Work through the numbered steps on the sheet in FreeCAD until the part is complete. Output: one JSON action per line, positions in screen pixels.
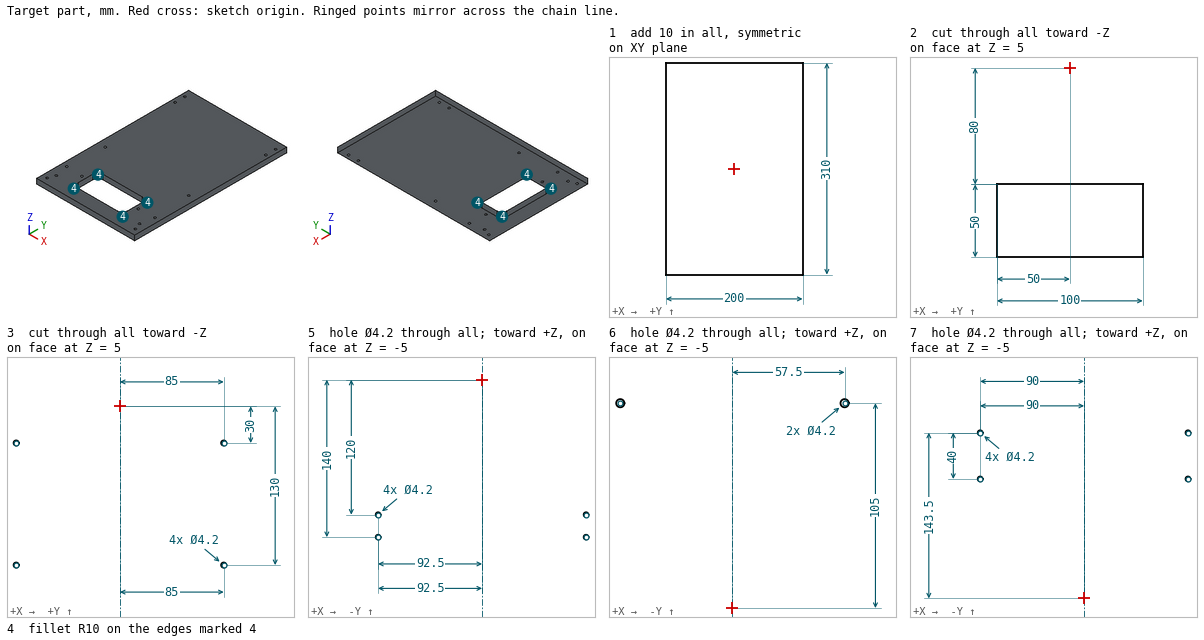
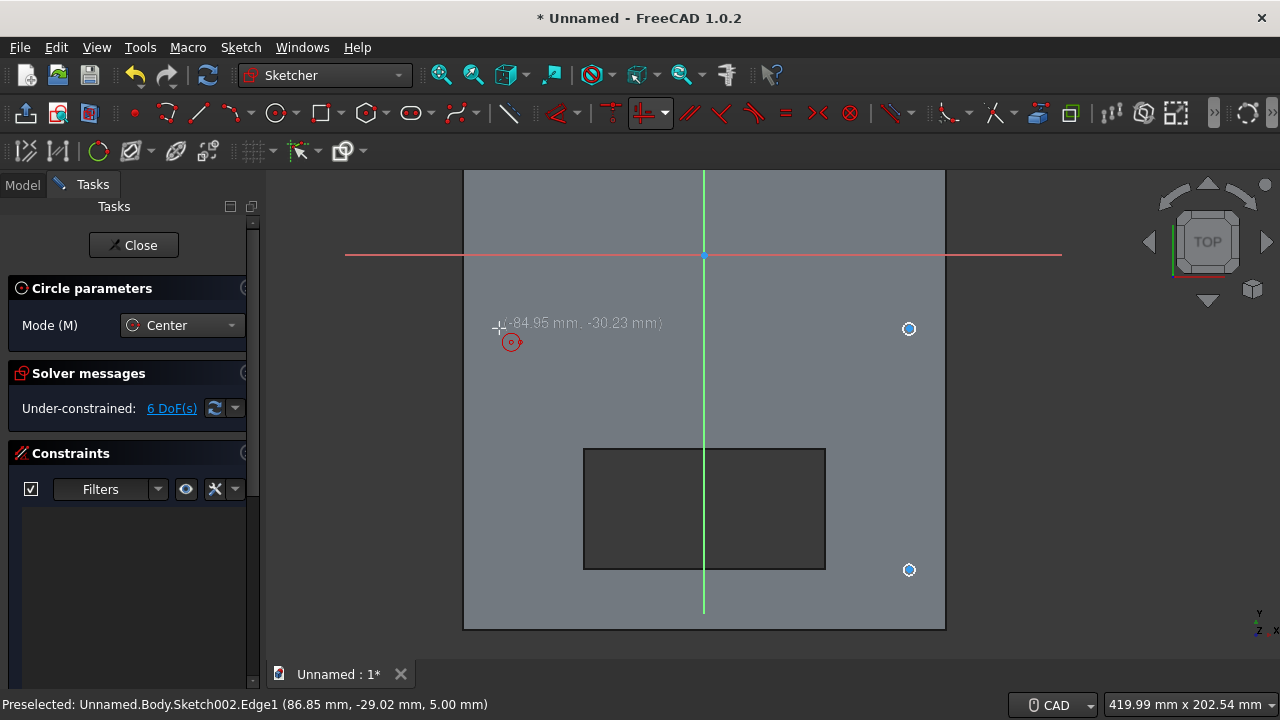
{"action": "left_click", "coordinate": [499, 328]}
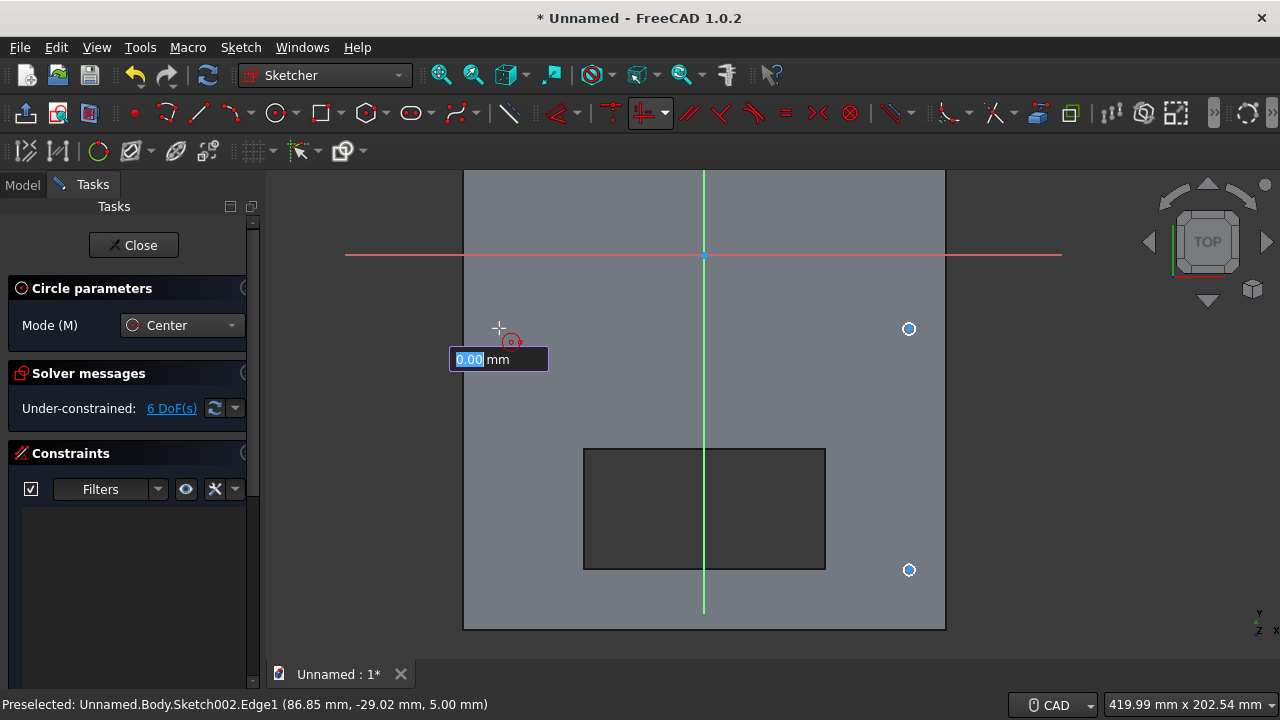
{"action": "scroll", "coordinate": [503, 324], "scroll_direction": "up", "scroll_amount": 6}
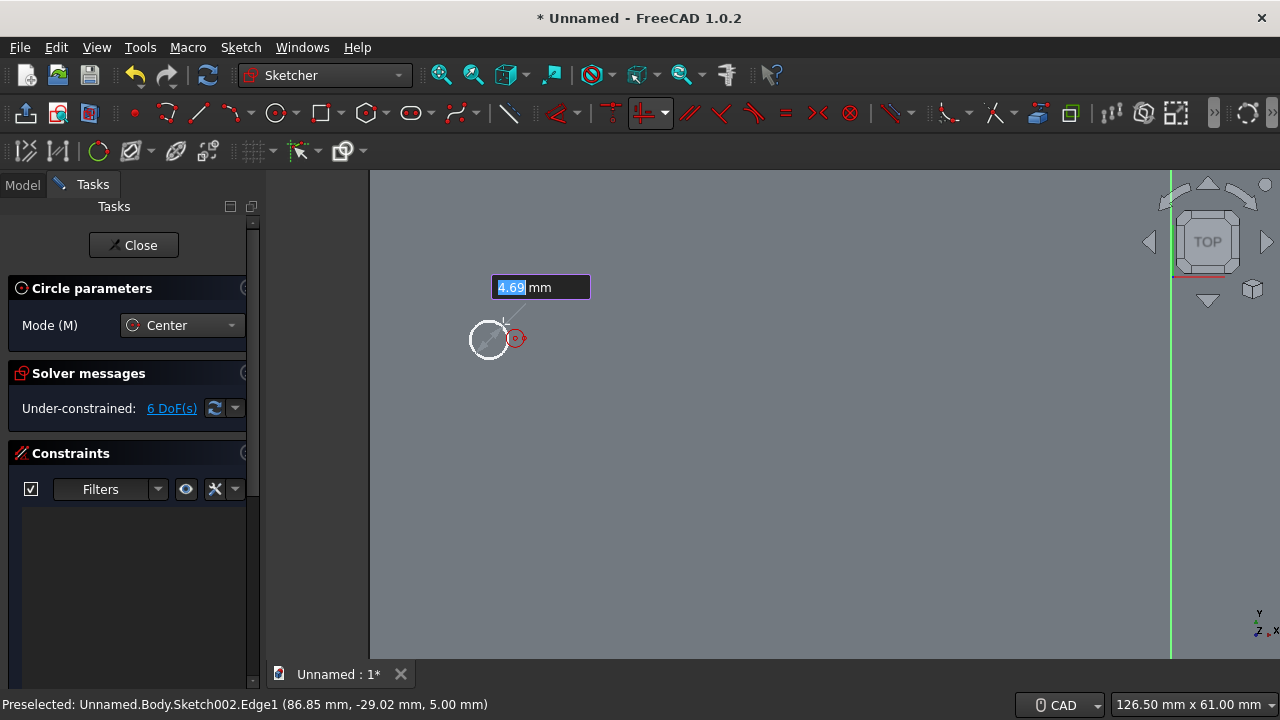
{"action": "left_click", "coordinate": [501, 324]}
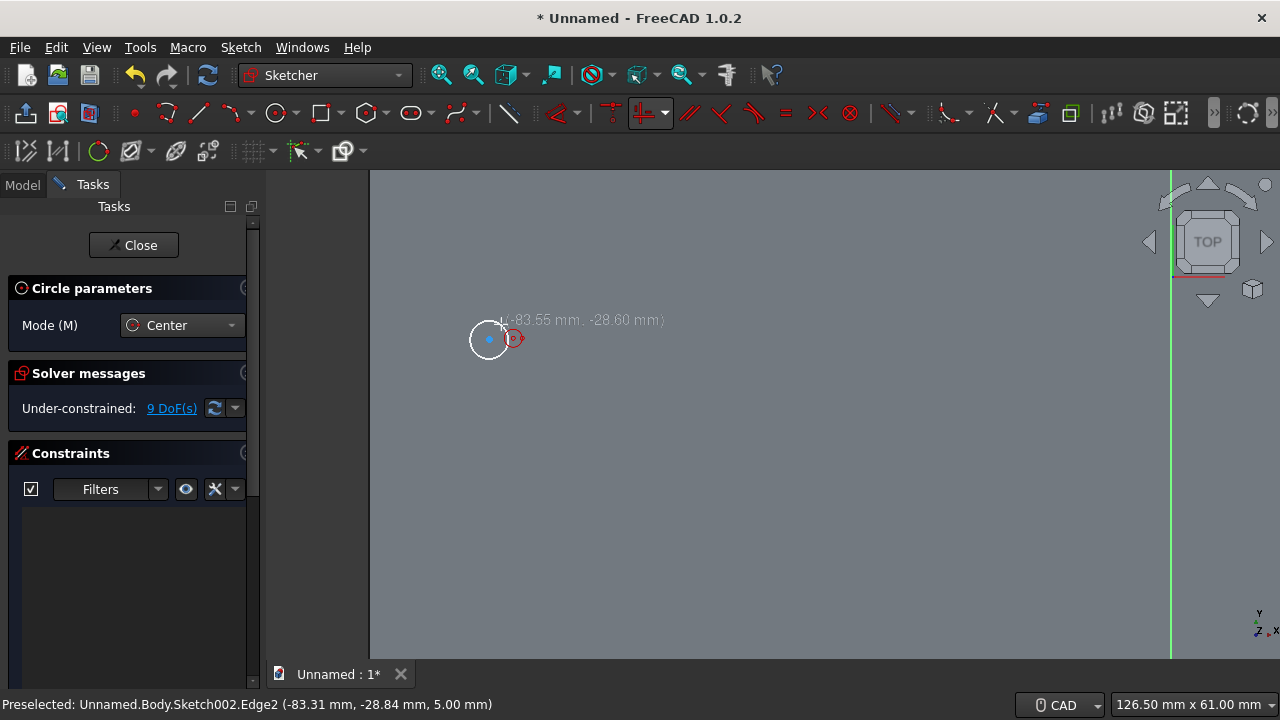
{"action": "scroll", "coordinate": [504, 324], "scroll_direction": "down", "scroll_amount": 6}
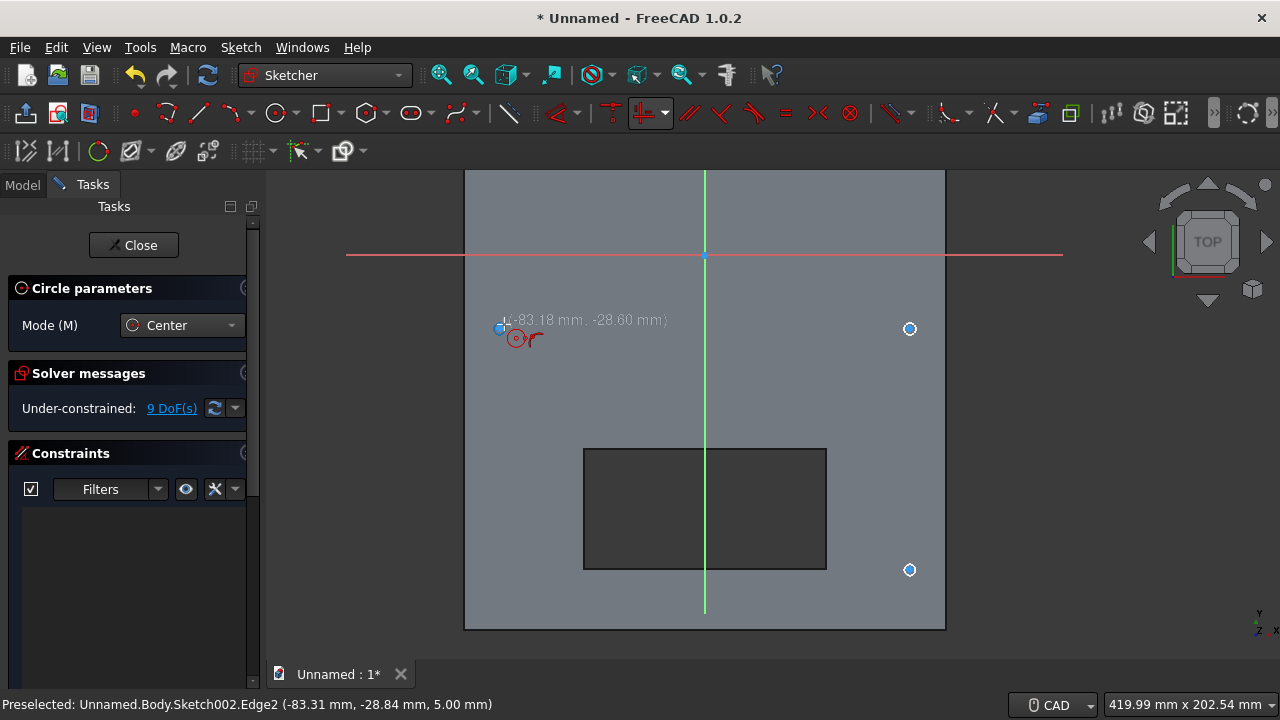
{"action": "scroll", "coordinate": [500, 569], "scroll_direction": "up", "scroll_amount": 8}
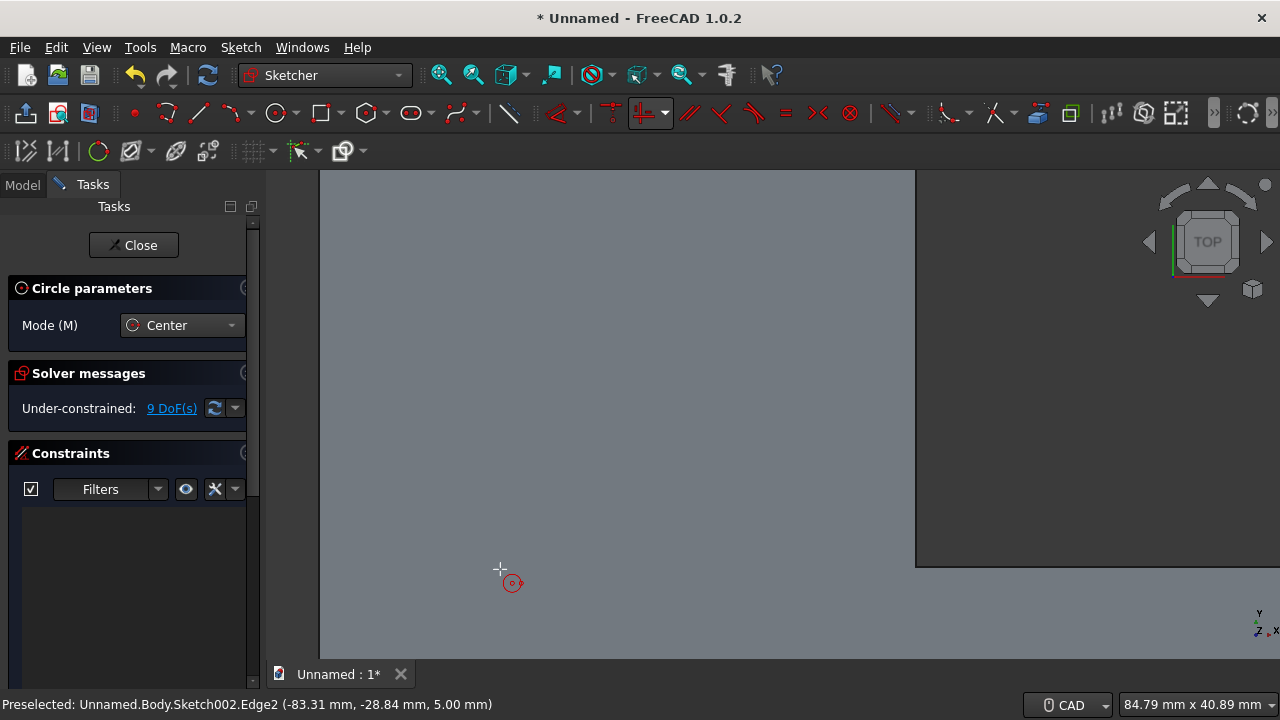
{"action": "scroll", "coordinate": [500, 569], "scroll_direction": "down", "scroll_amount": 8}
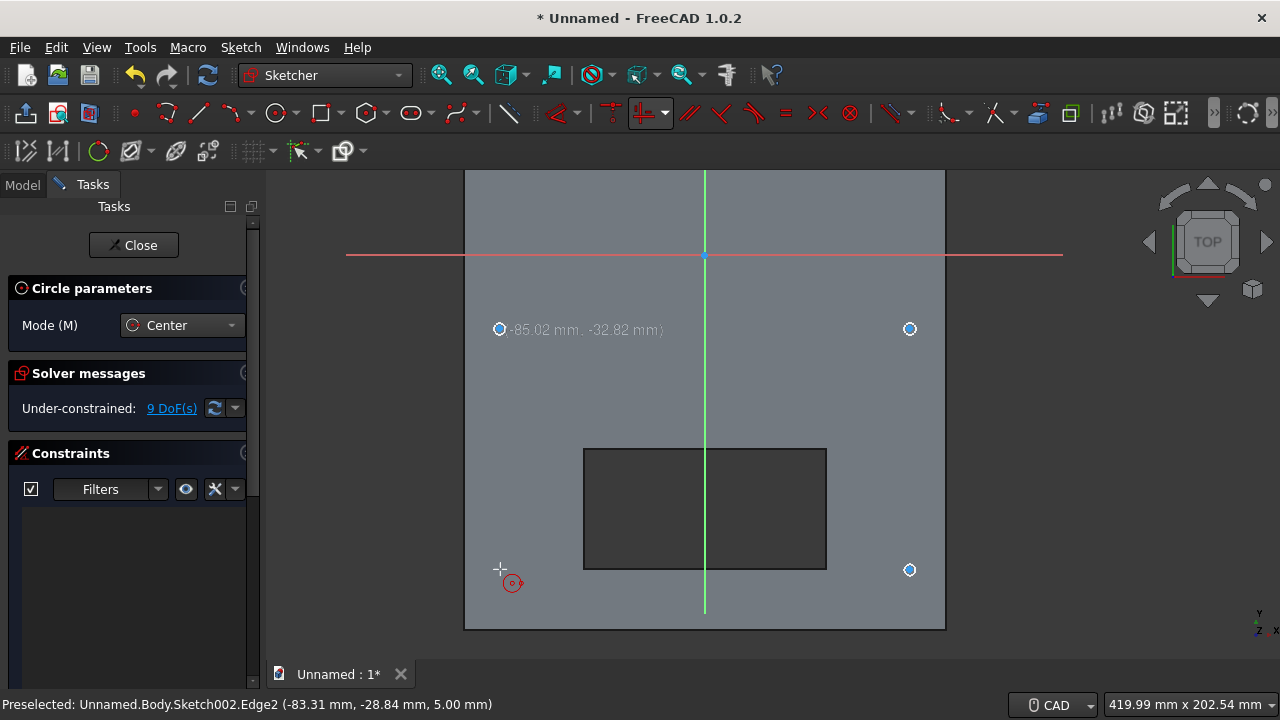
{"action": "left_click", "coordinate": [500, 569]}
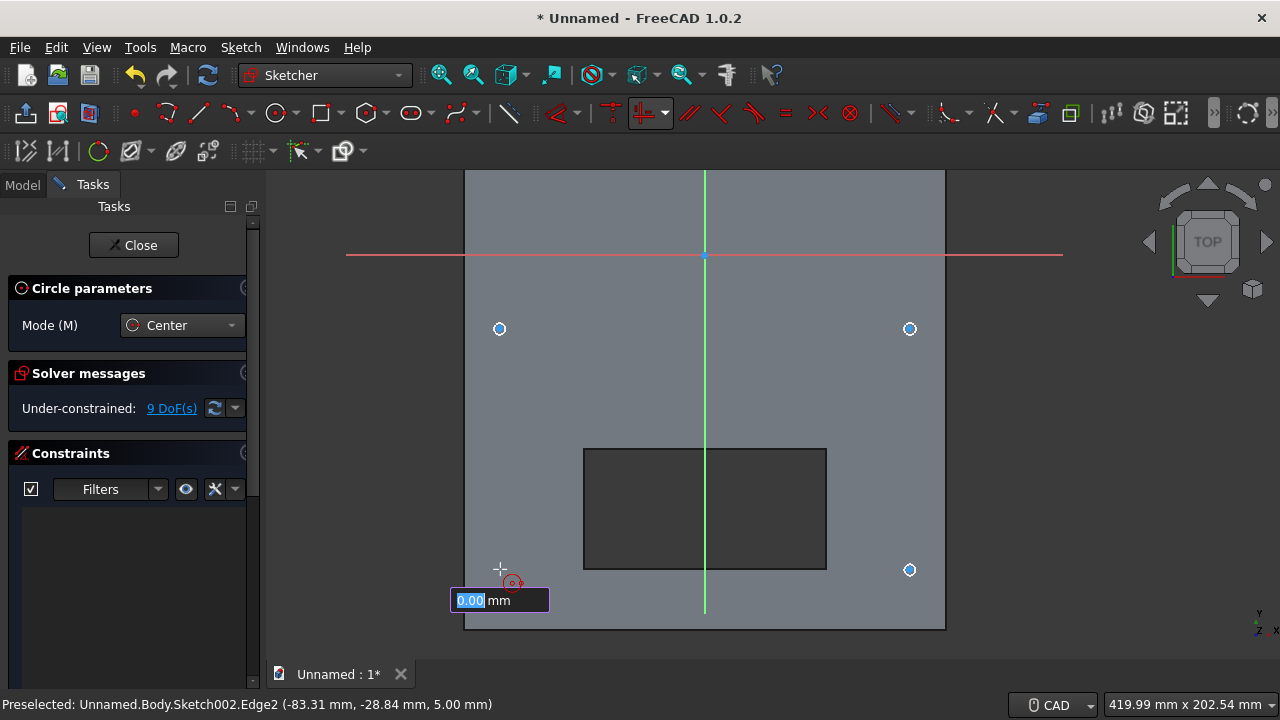
{"action": "scroll", "coordinate": [503, 566], "scroll_direction": "up", "scroll_amount": 6}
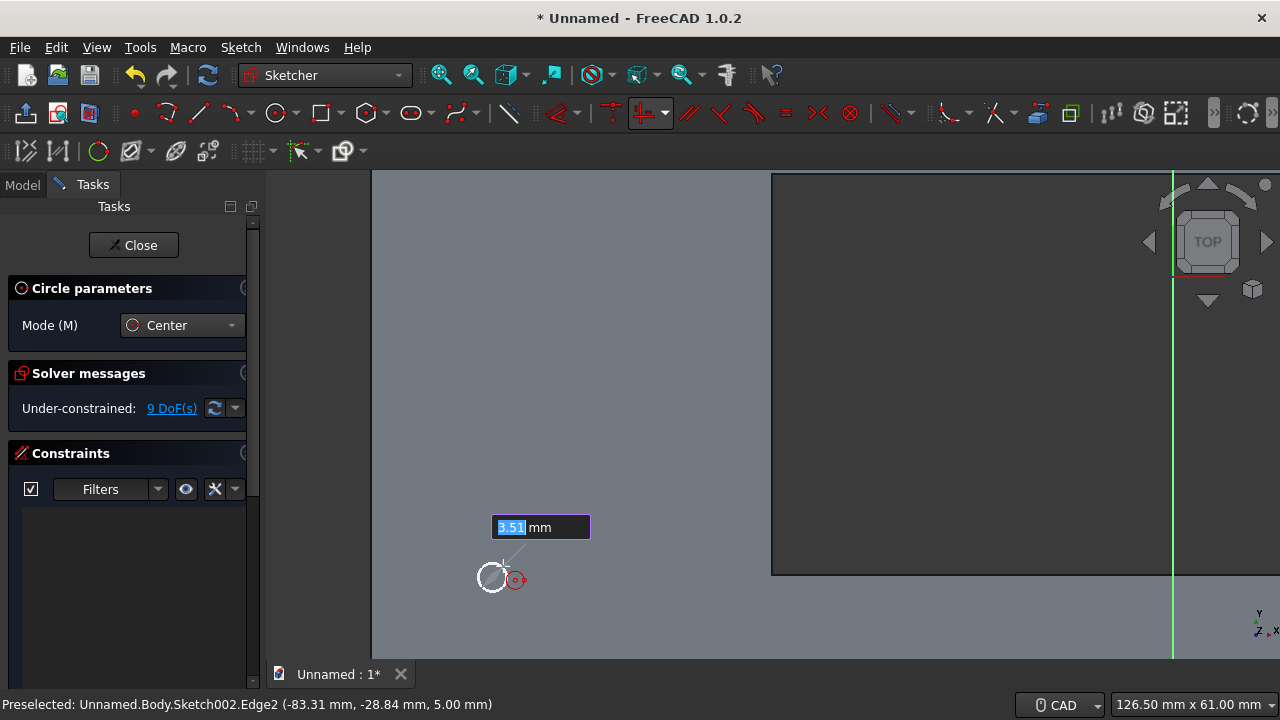
{"action": "left_click", "coordinate": [504, 563]}
{"action": "key", "text": "Escape"}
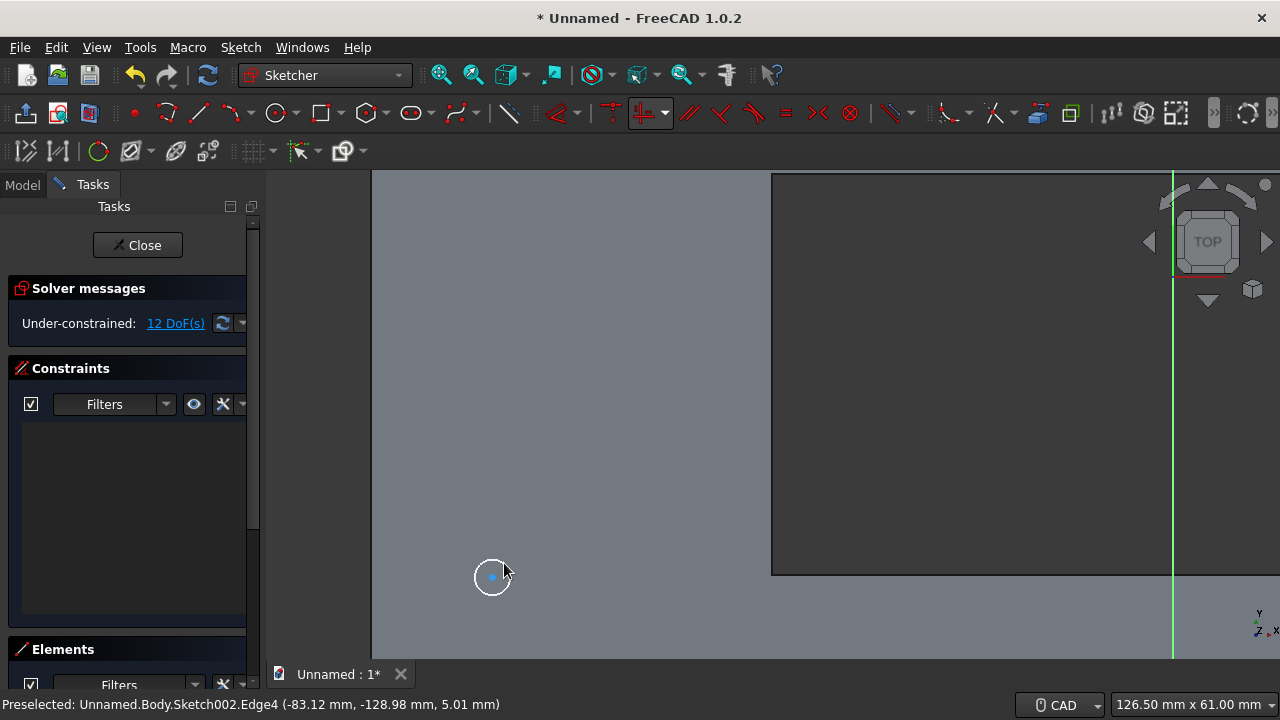
{"action": "scroll", "coordinate": [503, 566], "scroll_direction": "down", "scroll_amount": 6}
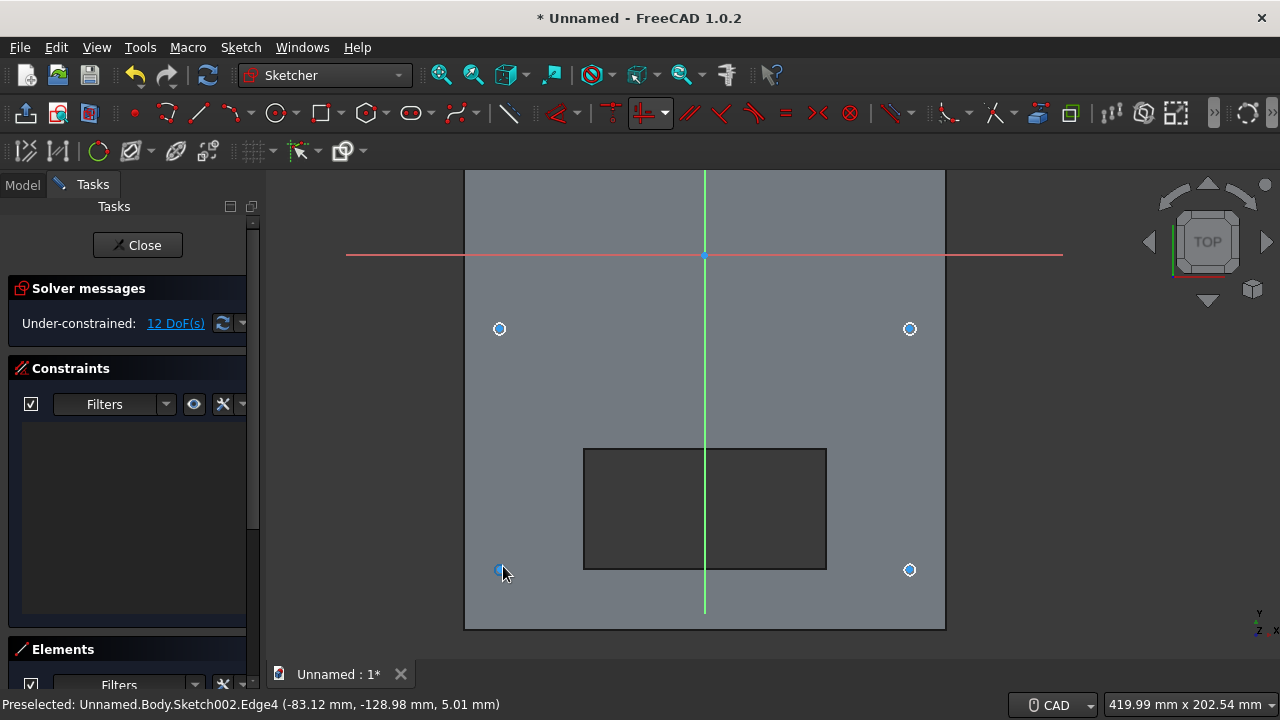
{"action": "scroll", "coordinate": [914, 566], "scroll_direction": "up", "scroll_amount": 5}